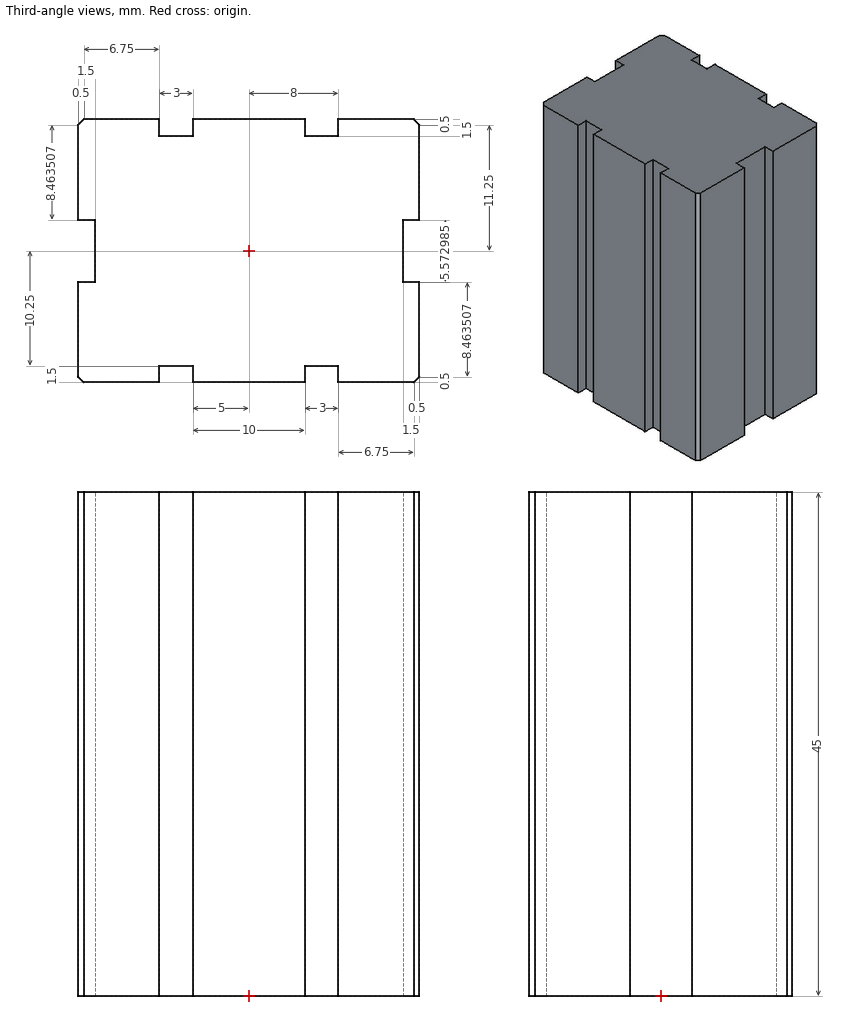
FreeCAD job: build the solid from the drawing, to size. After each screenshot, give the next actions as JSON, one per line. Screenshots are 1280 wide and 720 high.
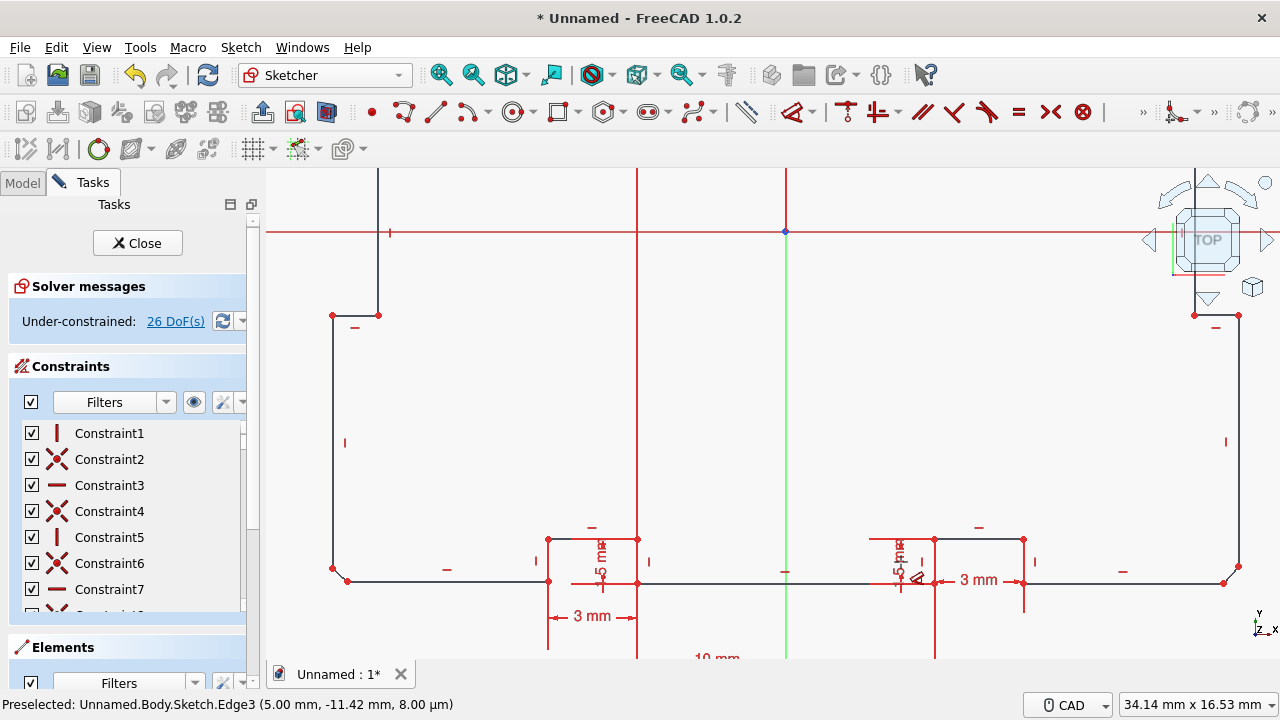
{"action": "left_click", "coordinate": [1024, 553]}
{"action": "left_click", "coordinate": [1058, 562]}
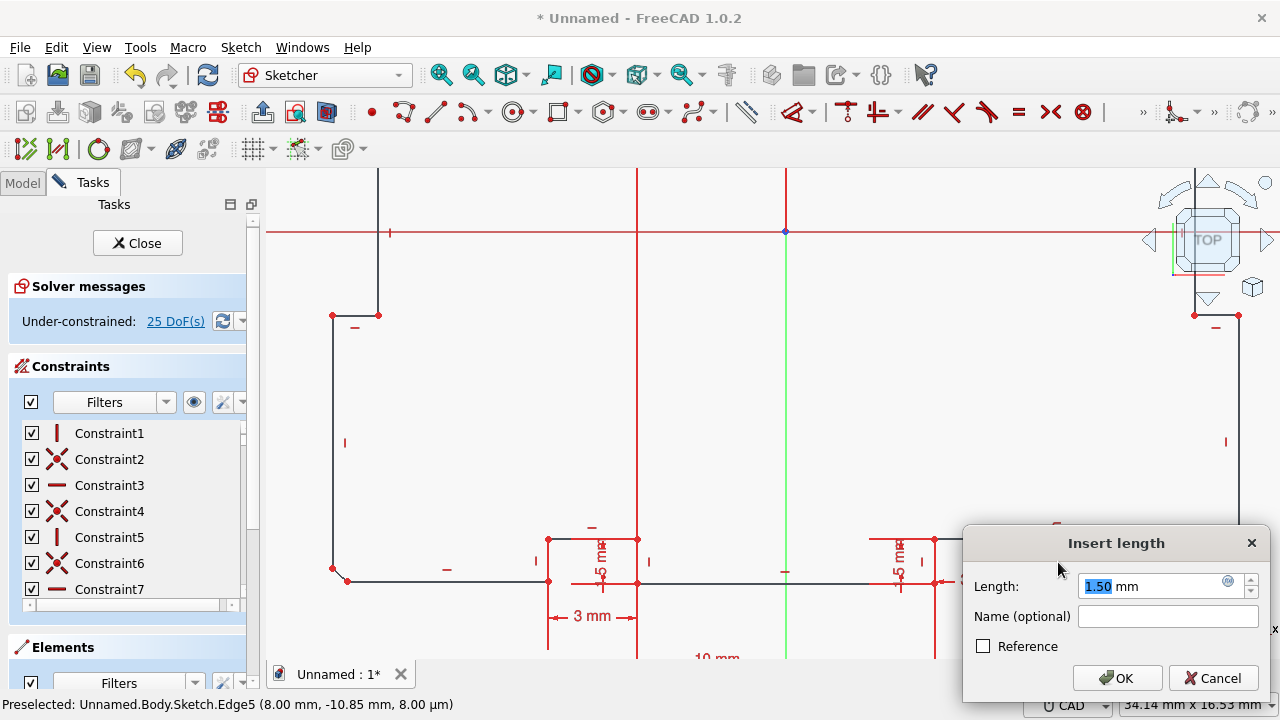
{"action": "type", "text": "1.5"}
{"action": "key", "text": "Return"}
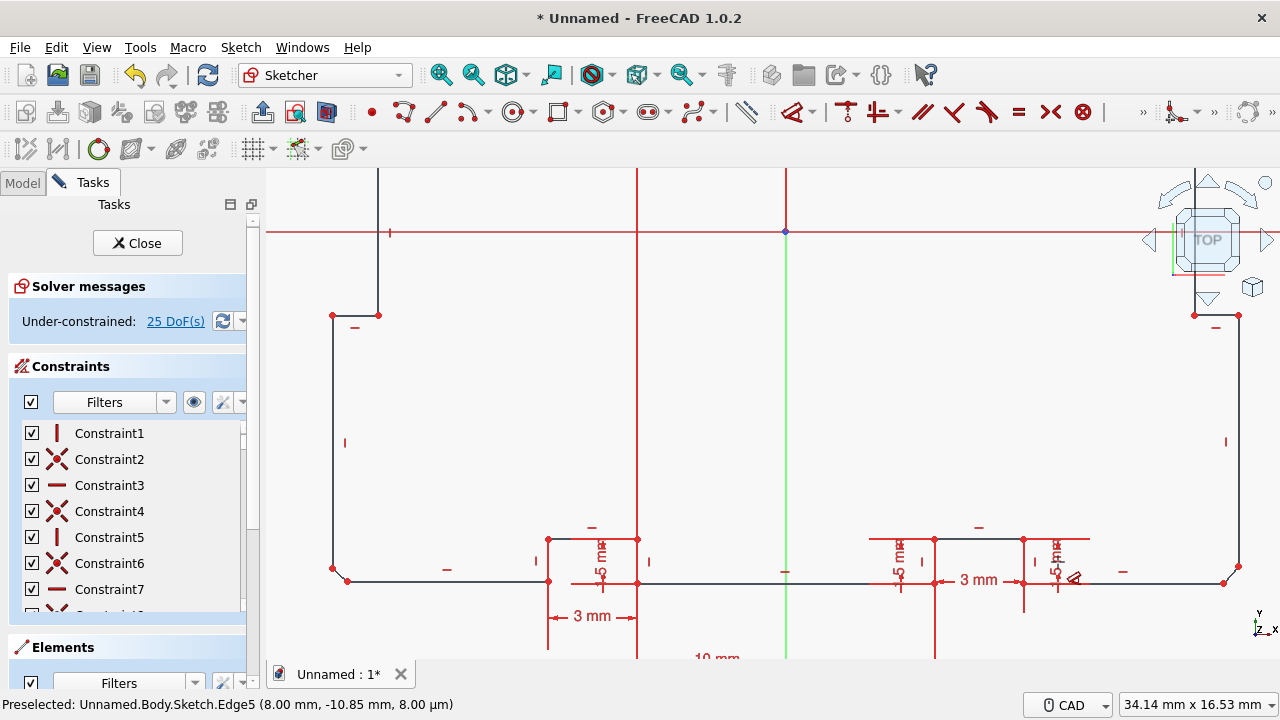
{"action": "scroll", "coordinate": [638, 562], "scroll_direction": "down", "scroll_amount": 4}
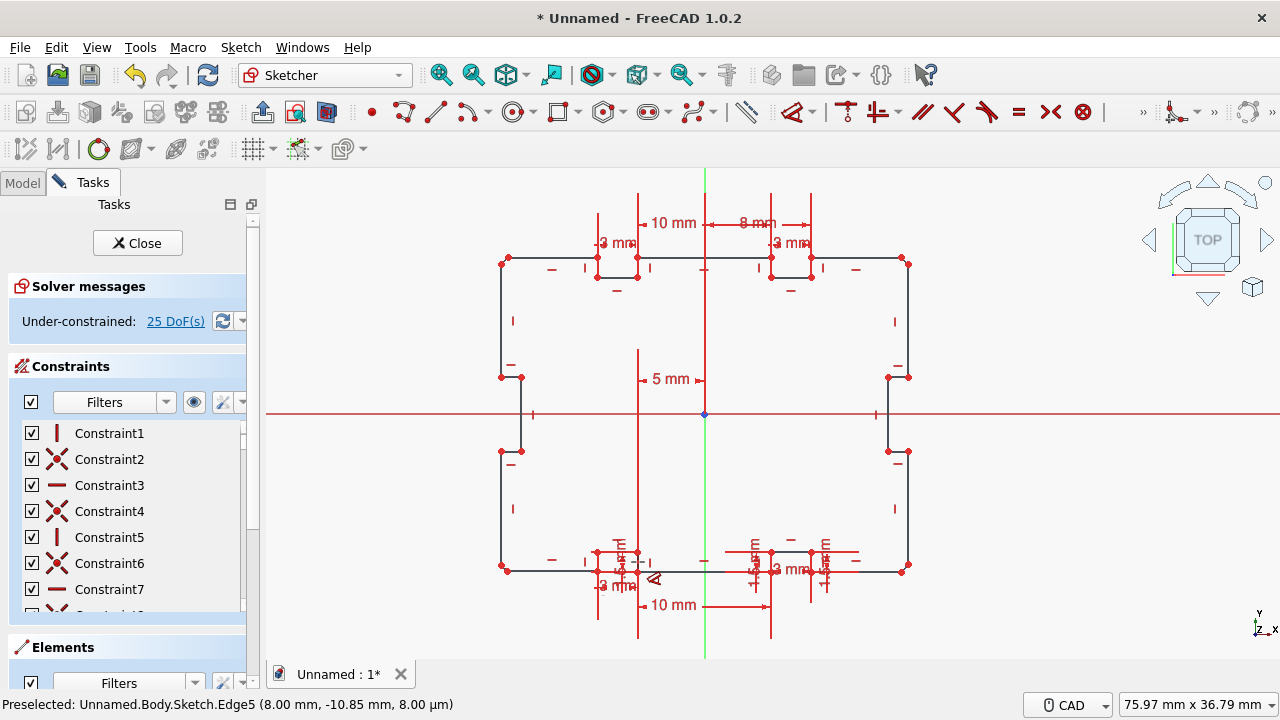
{"action": "scroll", "coordinate": [902, 452], "scroll_direction": "up", "scroll_amount": 5}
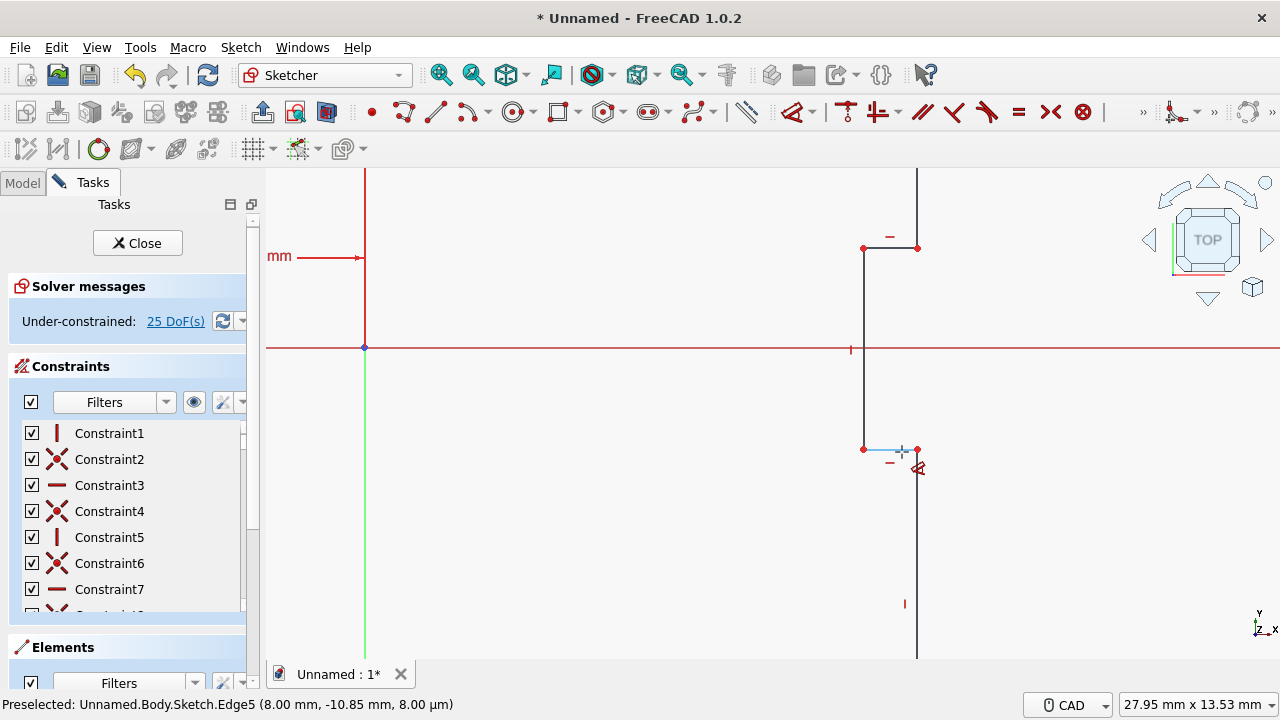
{"action": "left_click", "coordinate": [901, 450]}
{"action": "left_click", "coordinate": [891, 484]}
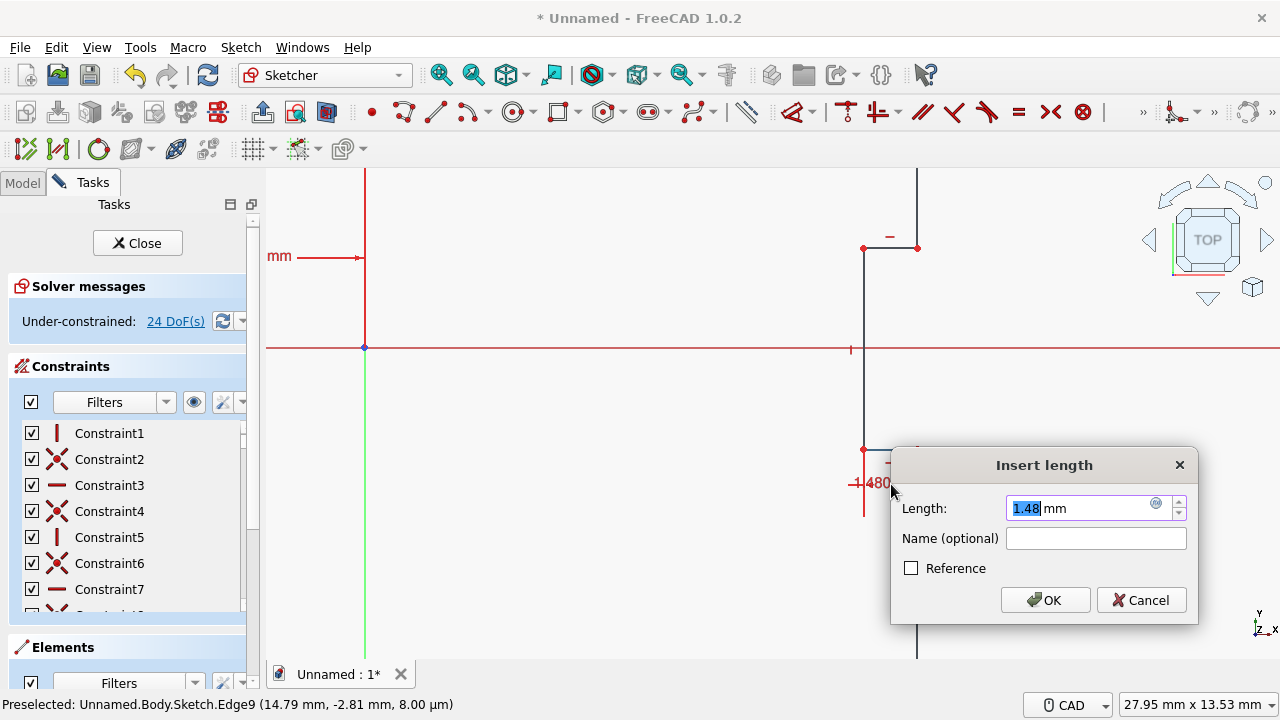
{"action": "type", "text": "1.5"}
{"action": "key", "text": "Return"}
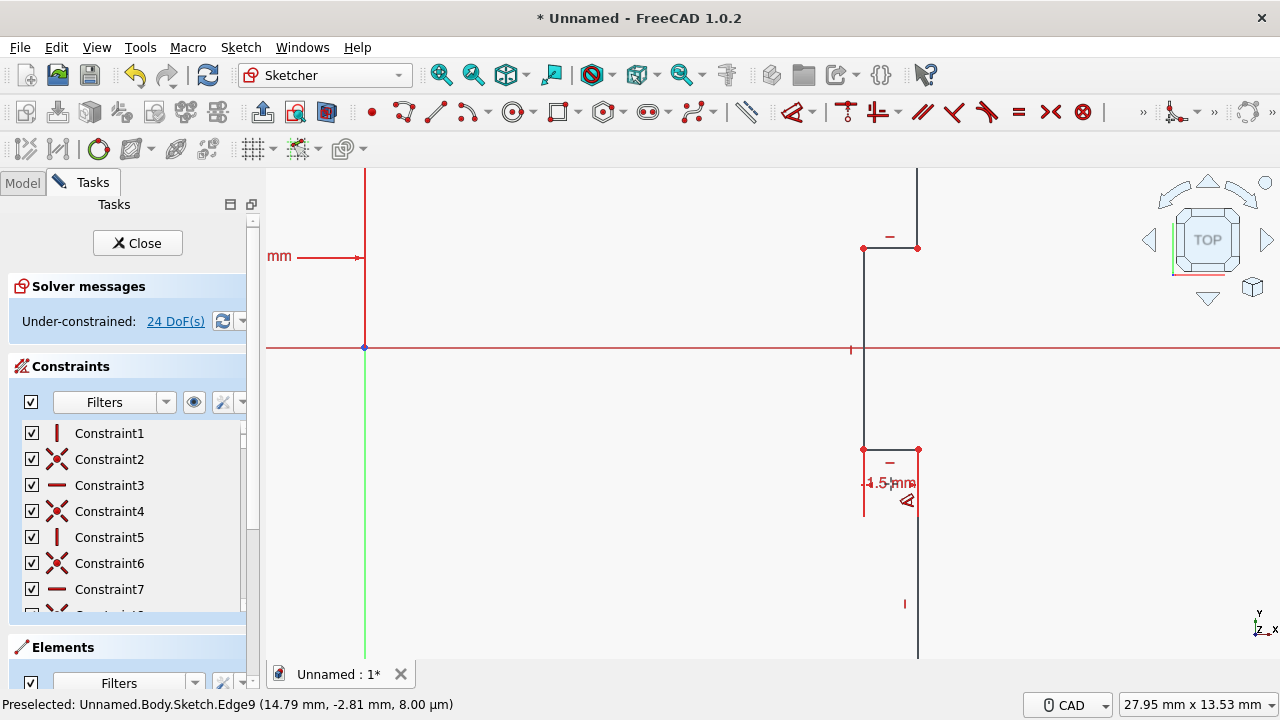
{"action": "left_click", "coordinate": [880, 248]}
{"action": "left_click", "coordinate": [891, 214]}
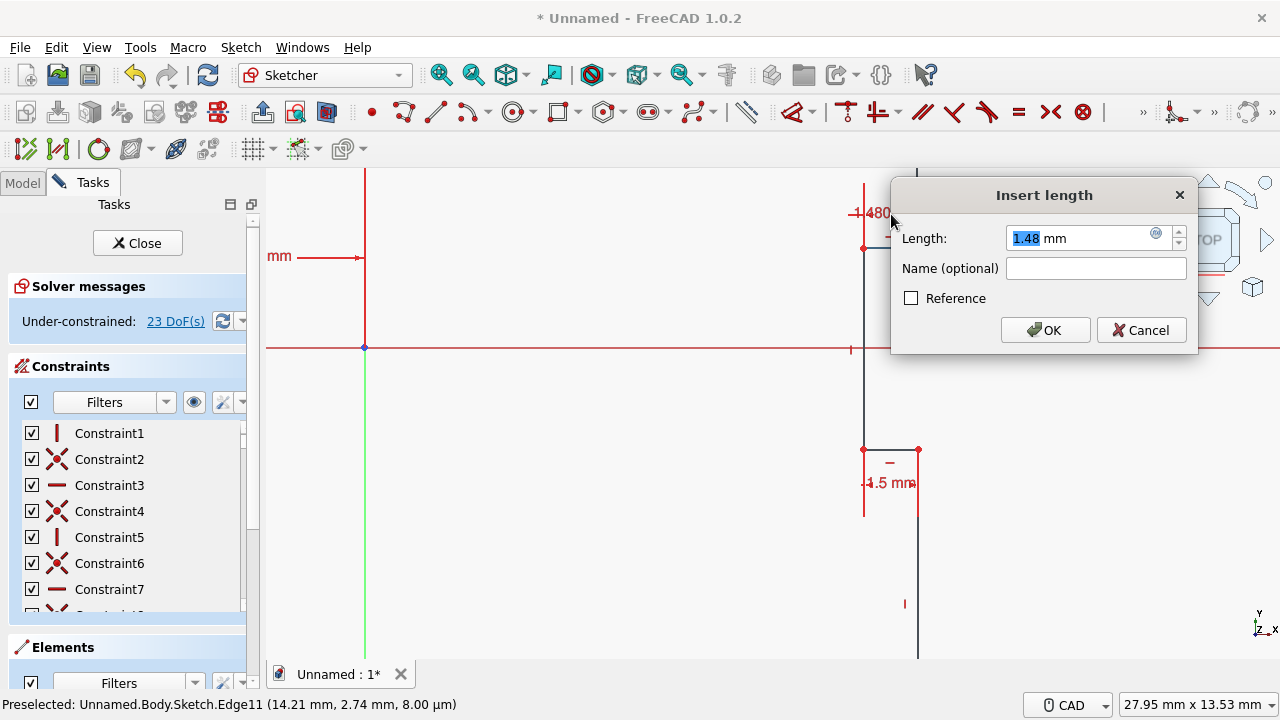
{"action": "type", "text": "1.5"}
{"action": "key", "text": "Return"}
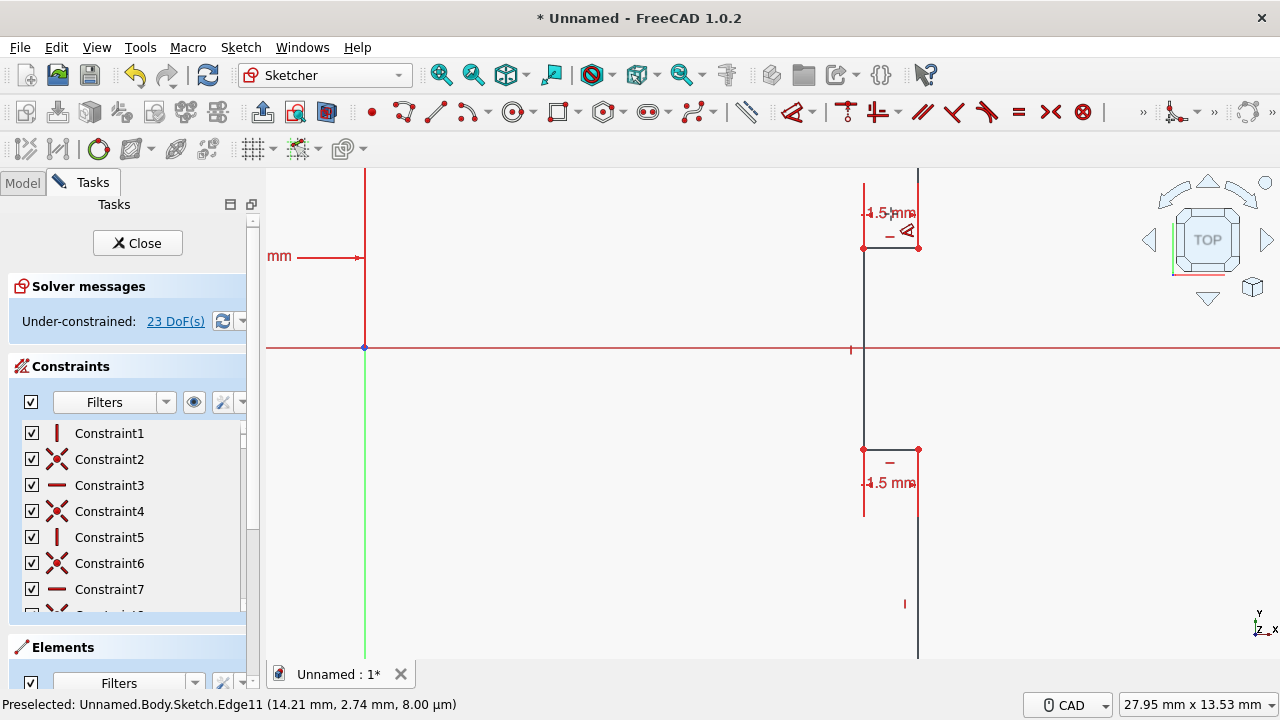
{"action": "scroll", "coordinate": [902, 452], "scroll_direction": "down", "scroll_amount": 5}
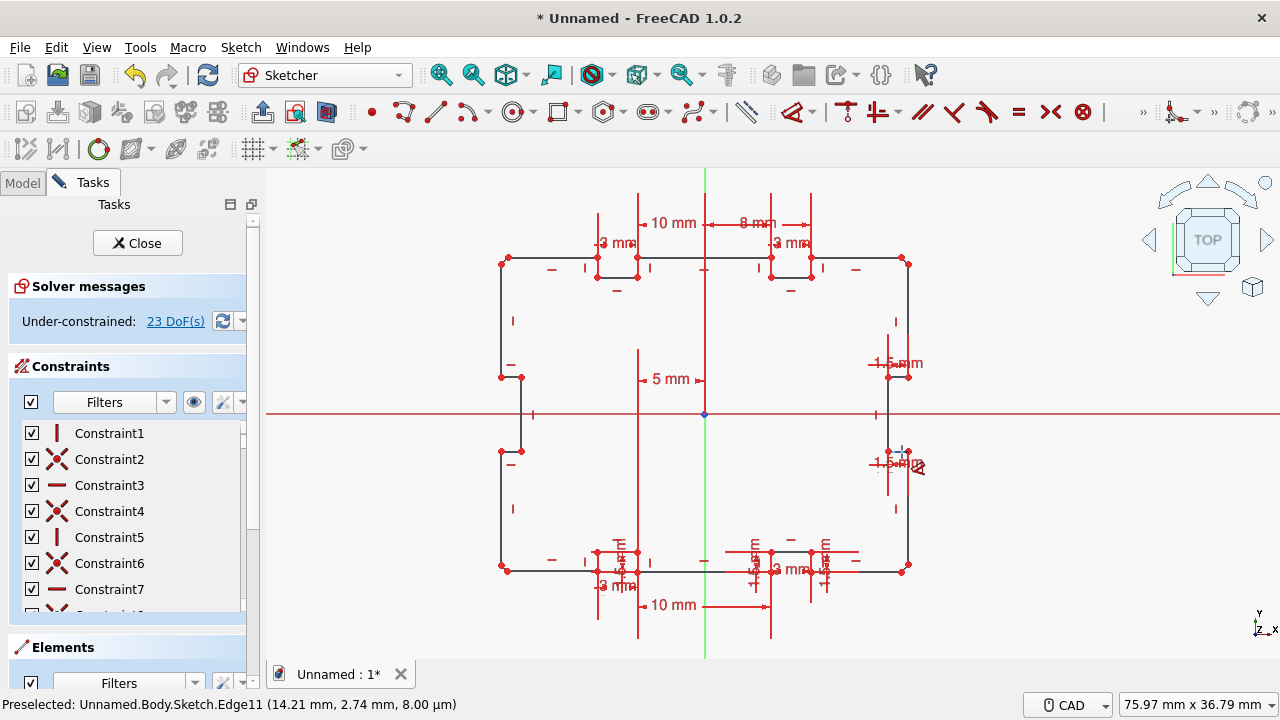
{"action": "scroll", "coordinate": [811, 264], "scroll_direction": "up", "scroll_amount": 5}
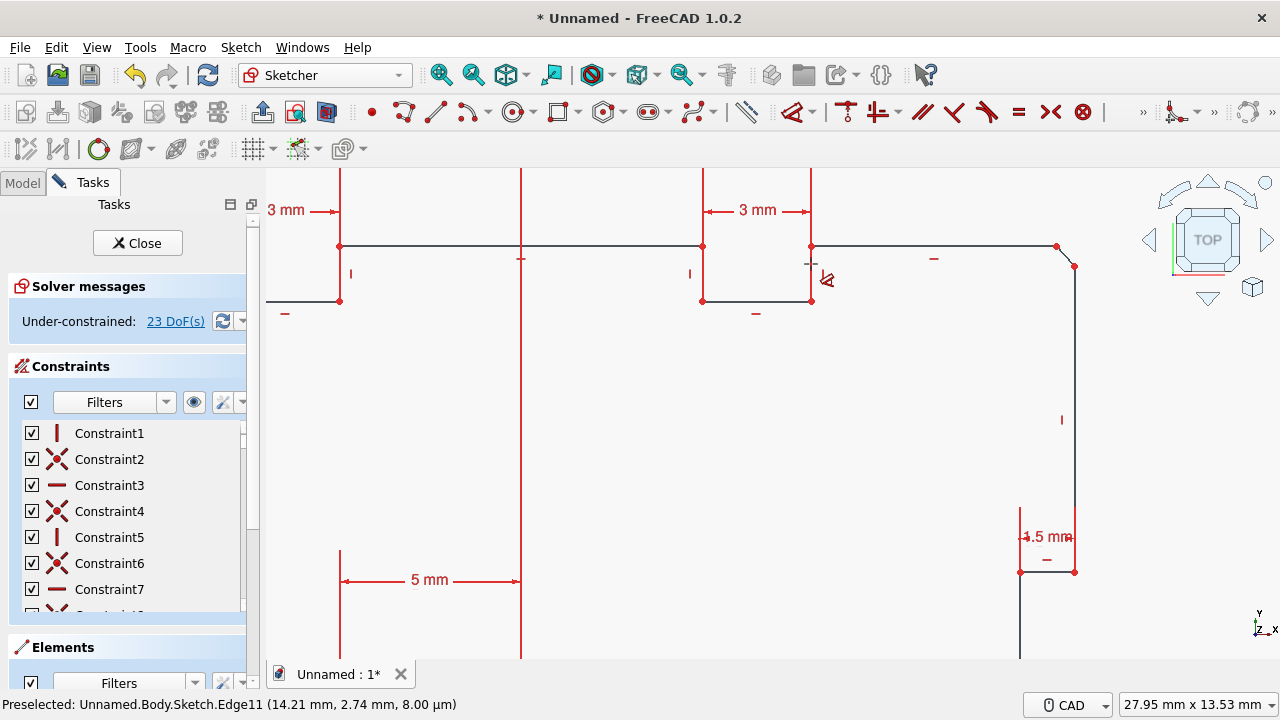
{"action": "left_click", "coordinate": [811, 263]}
{"action": "left_click", "coordinate": [845, 274]}